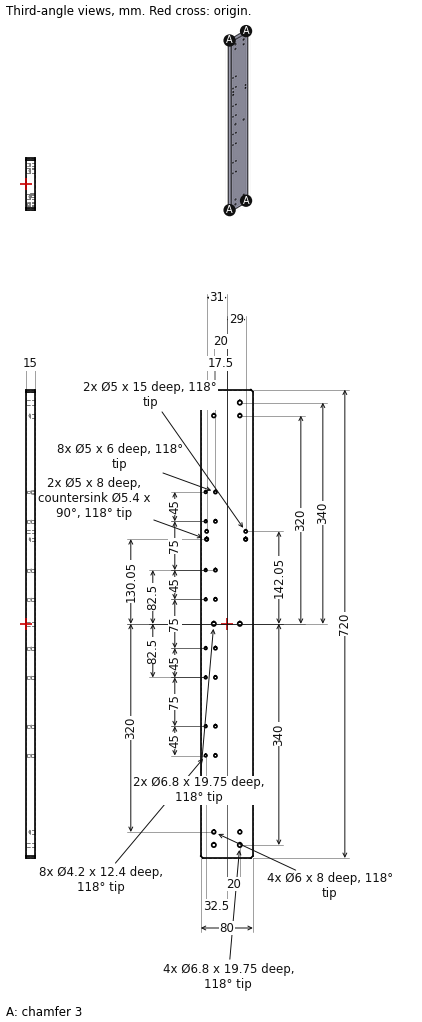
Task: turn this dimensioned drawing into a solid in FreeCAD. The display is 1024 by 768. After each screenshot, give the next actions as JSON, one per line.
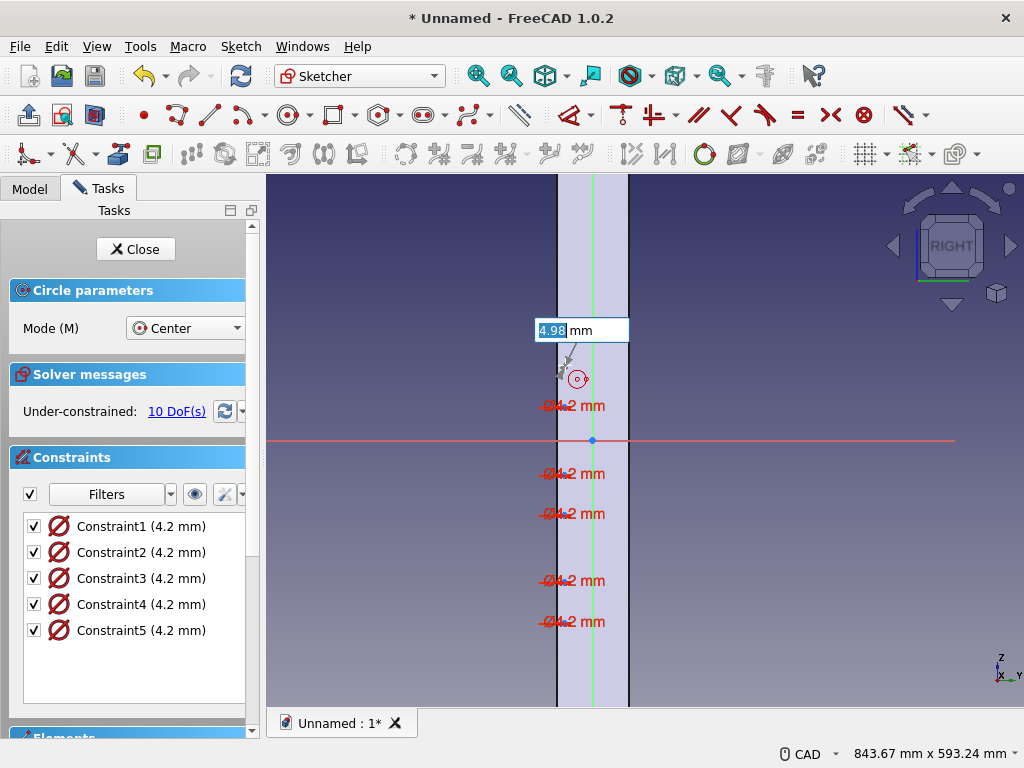
{"action": "type", "text": "4.2"}
{"action": "key", "text": "Return"}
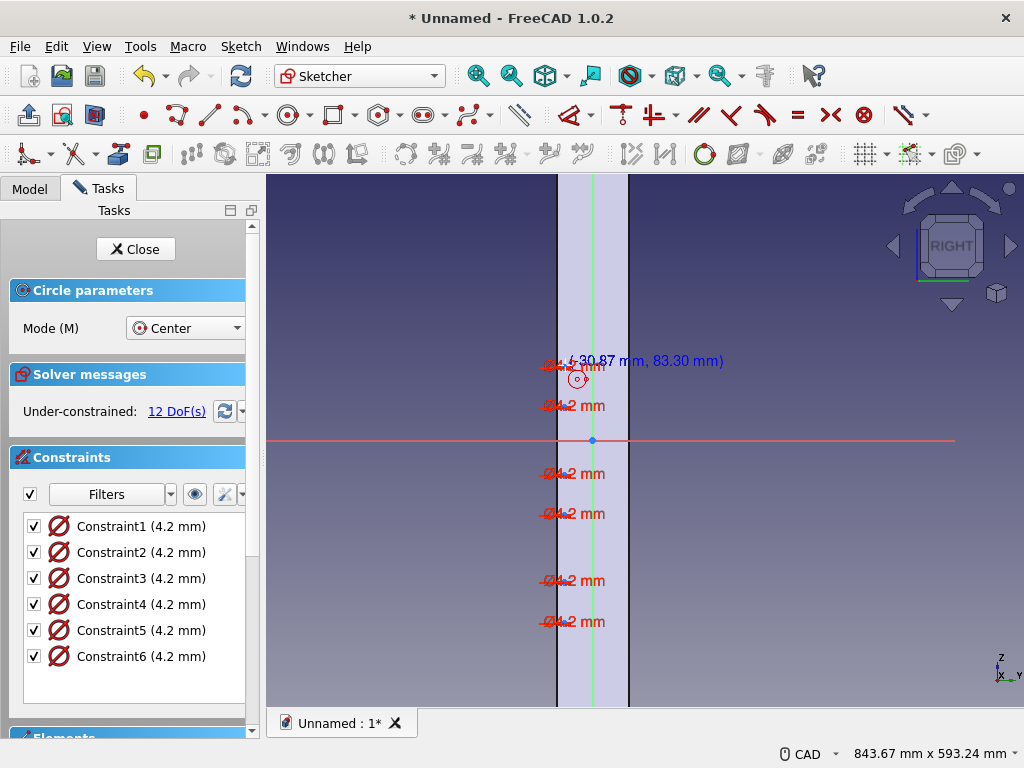
{"action": "scroll", "coordinate": [564, 299], "scroll_direction": "up", "scroll_amount": 13}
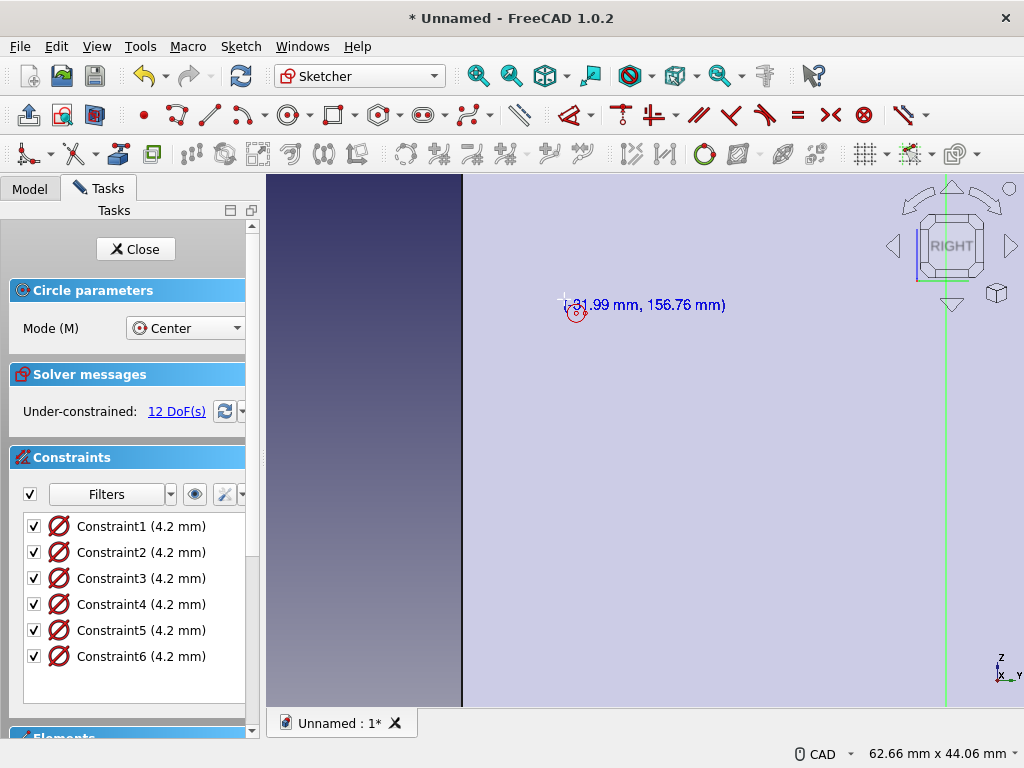
{"action": "scroll", "coordinate": [564, 299], "scroll_direction": "down", "scroll_amount": 13}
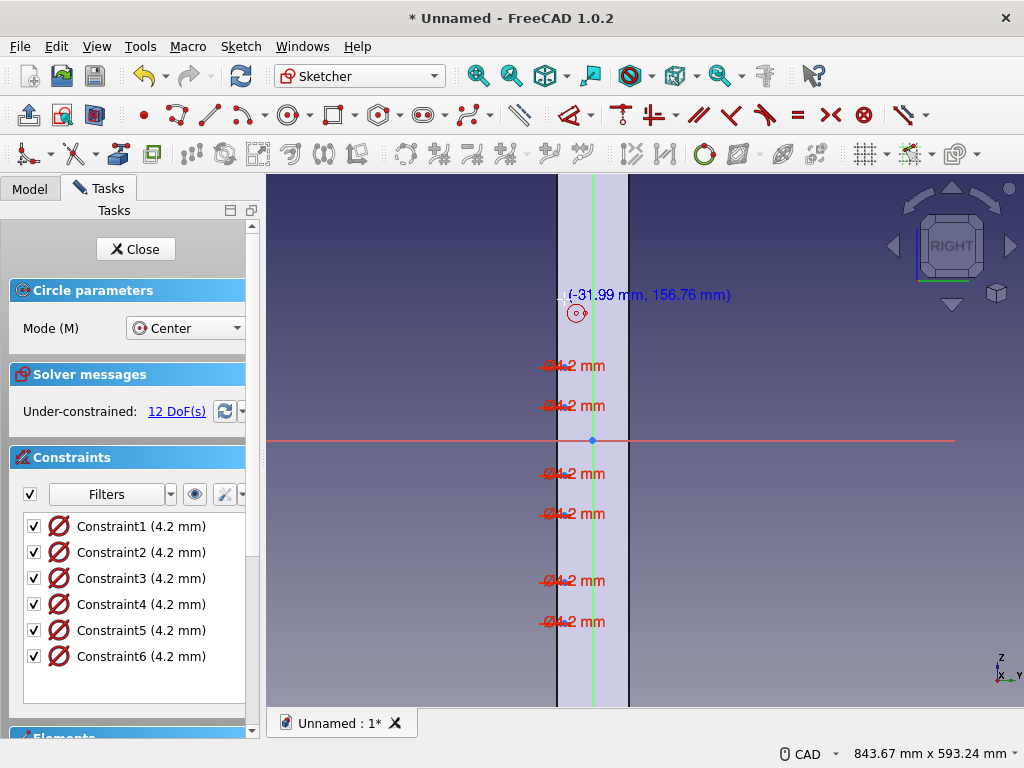
{"action": "left_click", "coordinate": [564, 299]}
{"action": "mouse_move", "coordinate": [565, 298]}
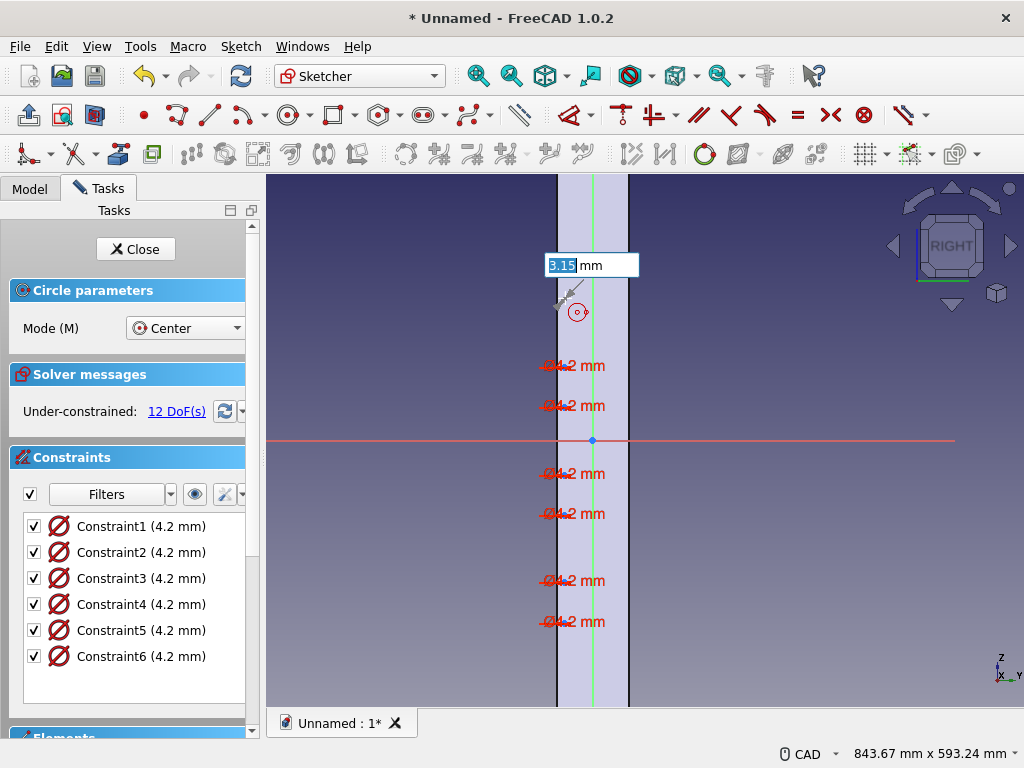
{"action": "type", "text": "4.2"}
{"action": "key", "text": "Return"}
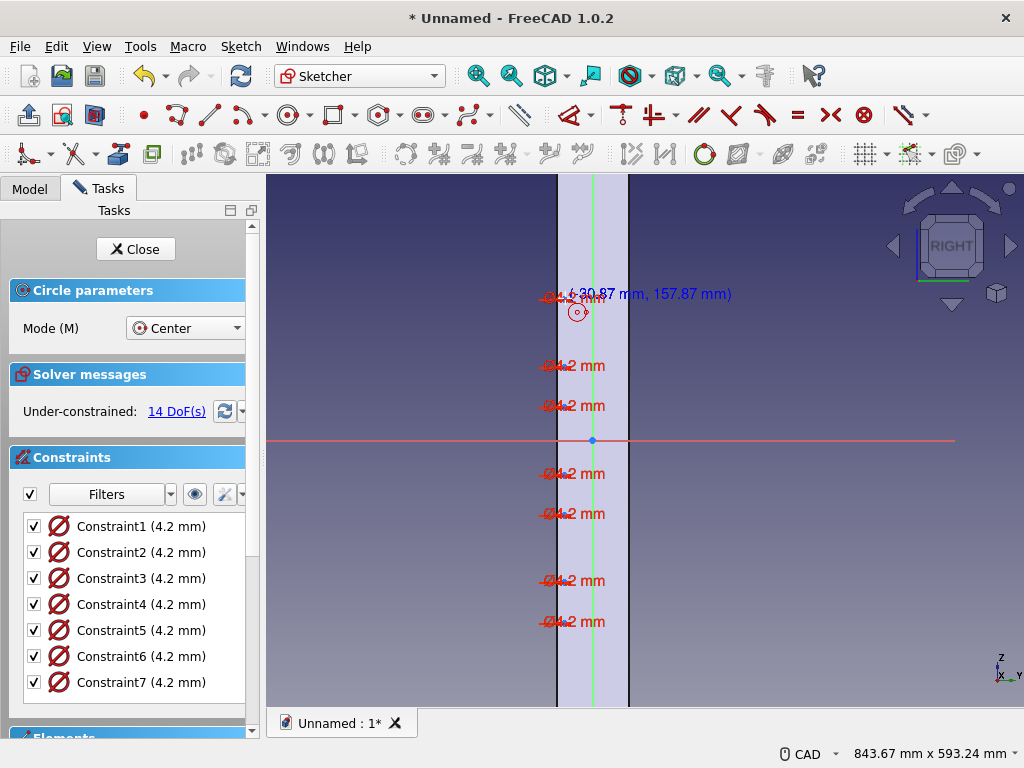
{"action": "scroll", "coordinate": [564, 259], "scroll_direction": "up", "scroll_amount": 13}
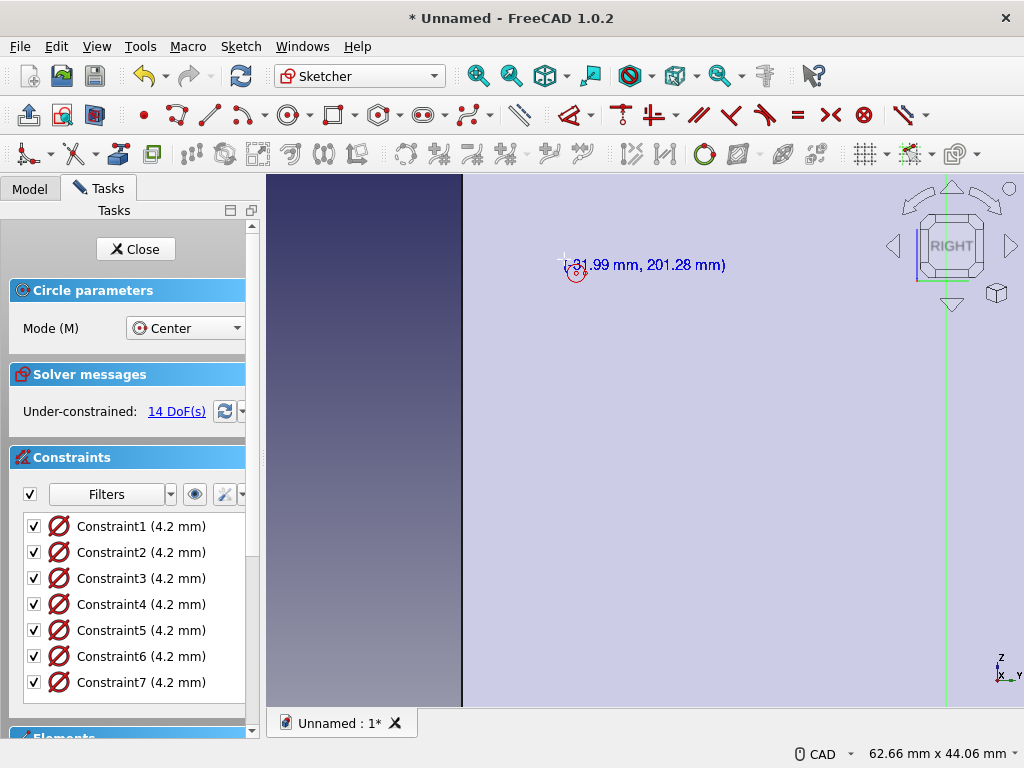
{"action": "scroll", "coordinate": [564, 259], "scroll_direction": "down", "scroll_amount": 13}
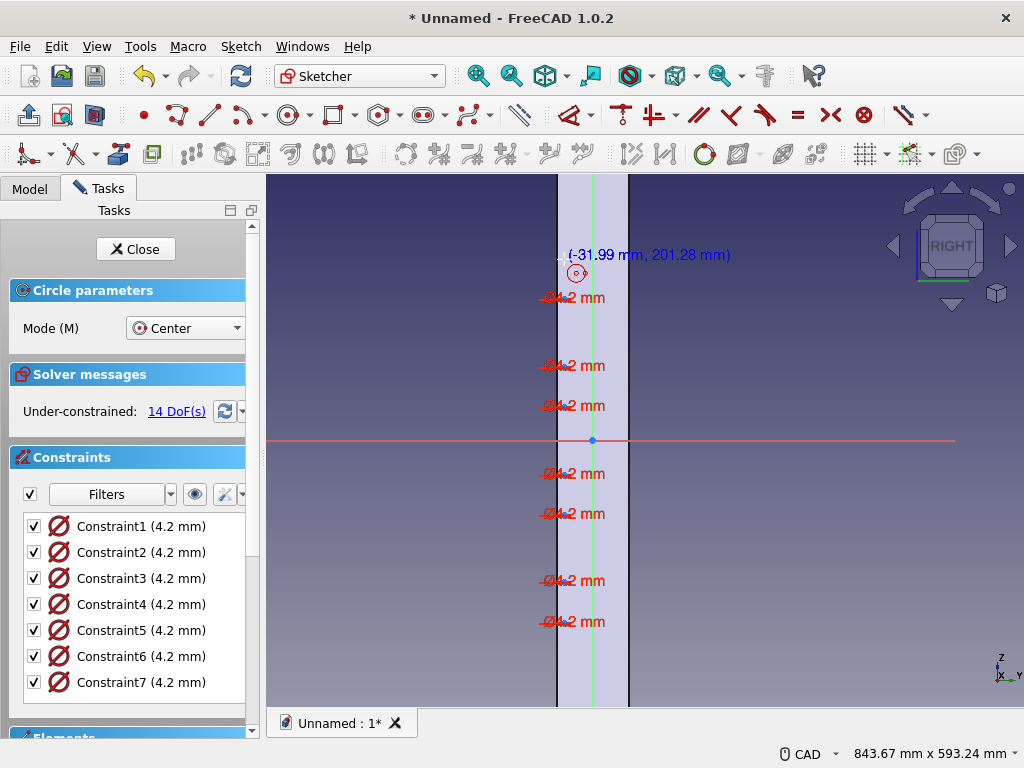
{"action": "left_click", "coordinate": [564, 259]}
{"action": "mouse_move", "coordinate": [565, 258]}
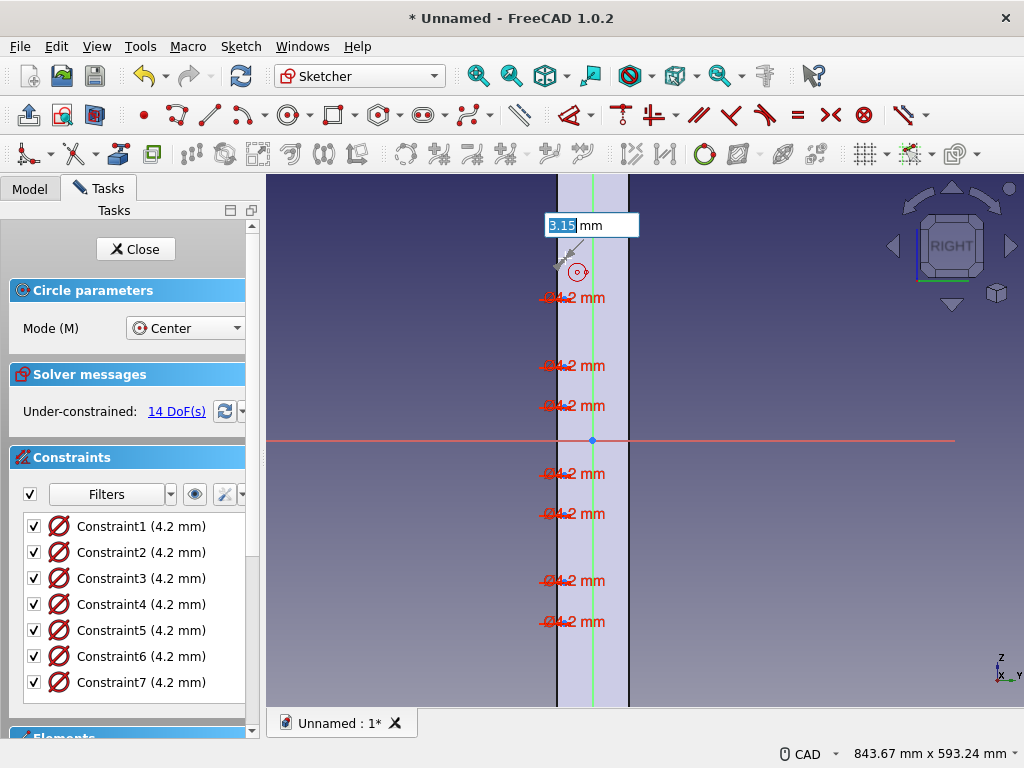
{"action": "type", "text": "4.2"}
{"action": "key", "text": "Return"}
{"action": "key", "text": "Escape"}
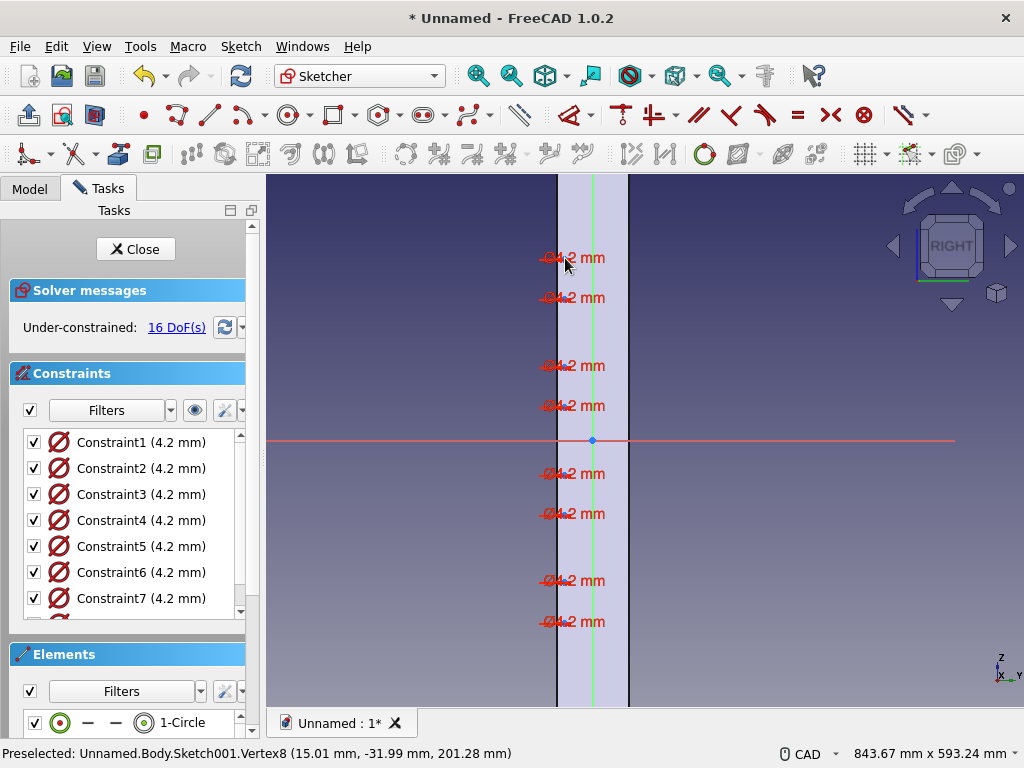
{"action": "left_click", "coordinate": [564, 624]}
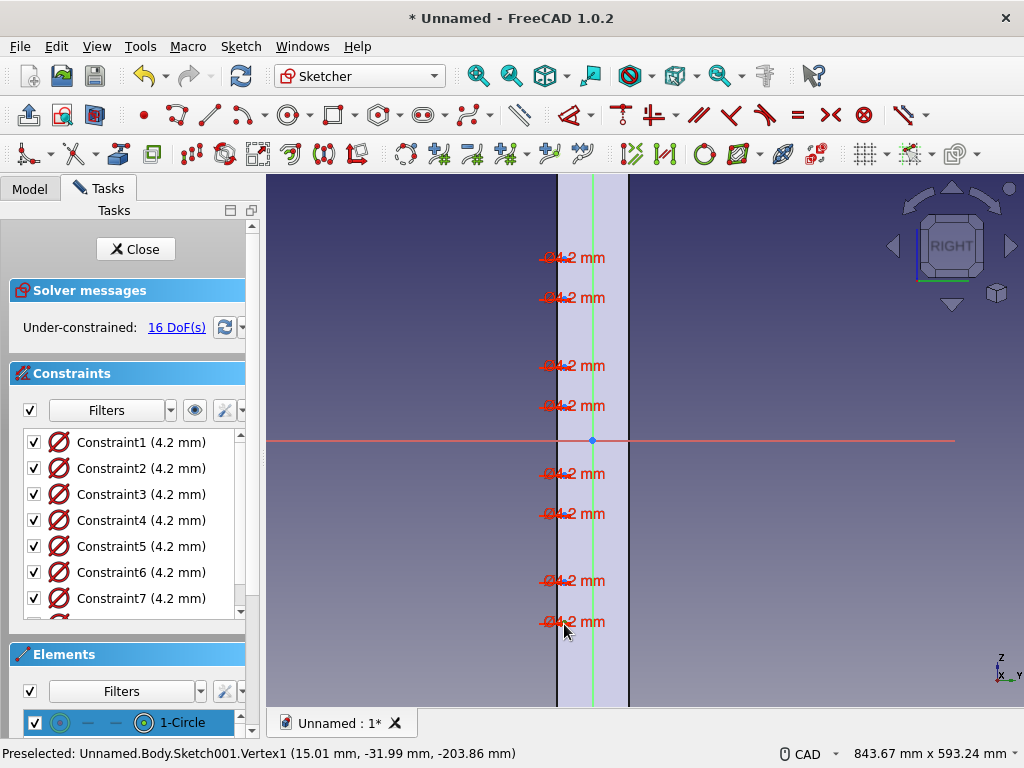
{"action": "left_click", "coordinate": [564, 583]}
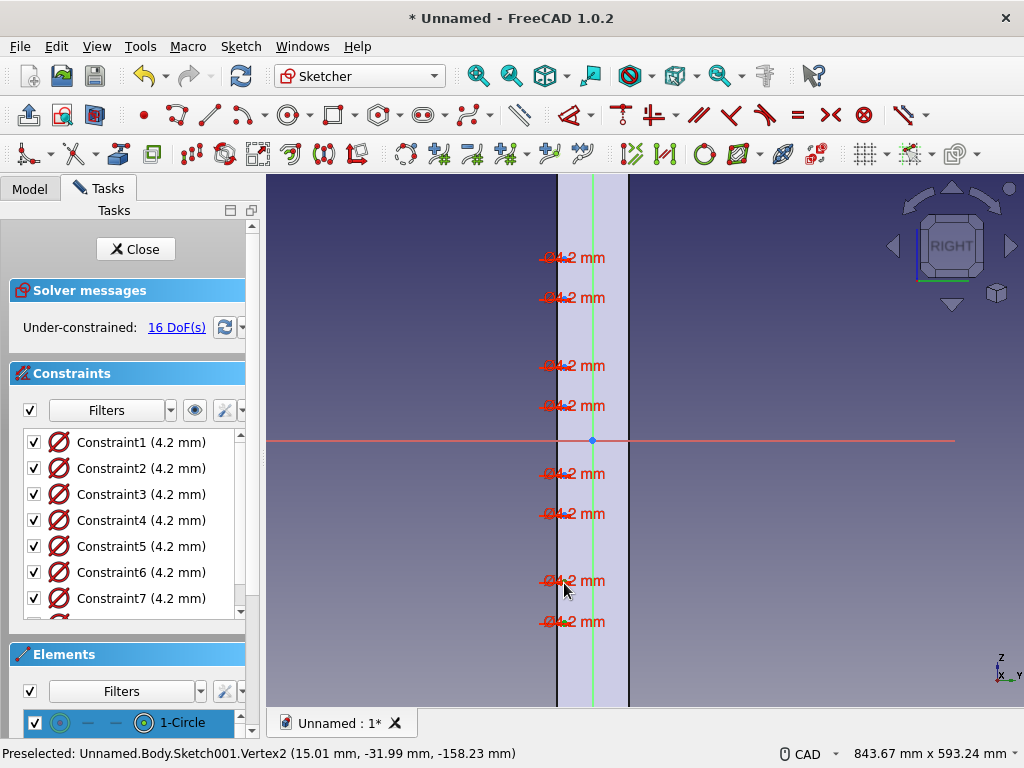
{"action": "left_click", "coordinate": [676, 116]}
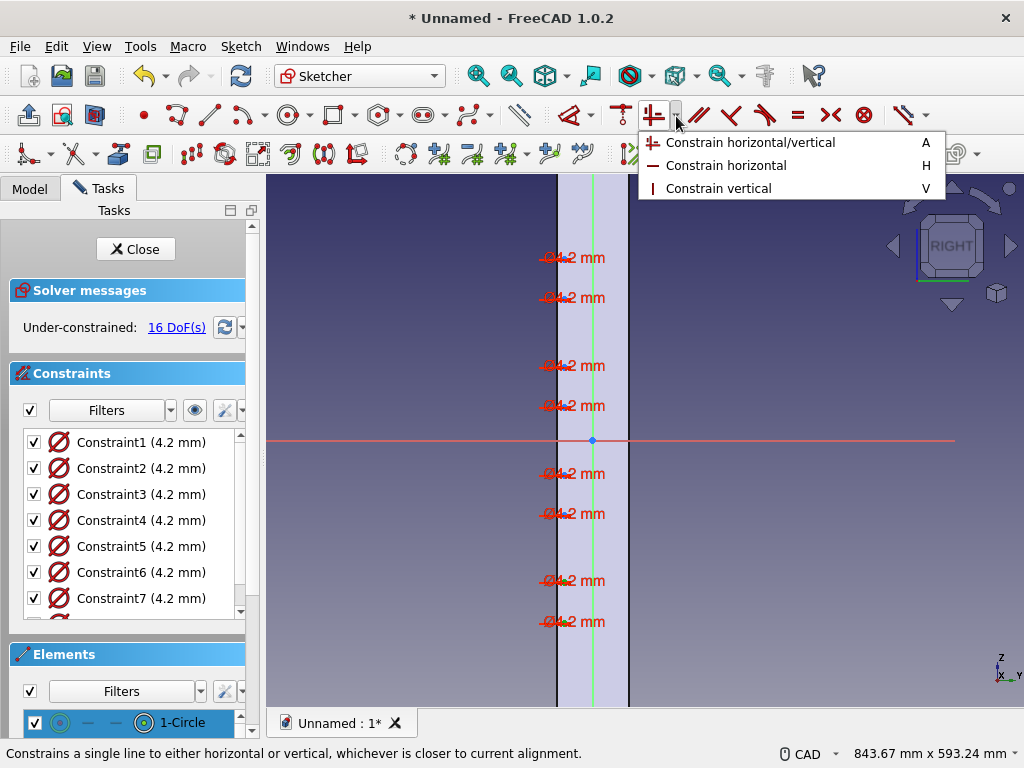
{"action": "left_click", "coordinate": [792, 188]}